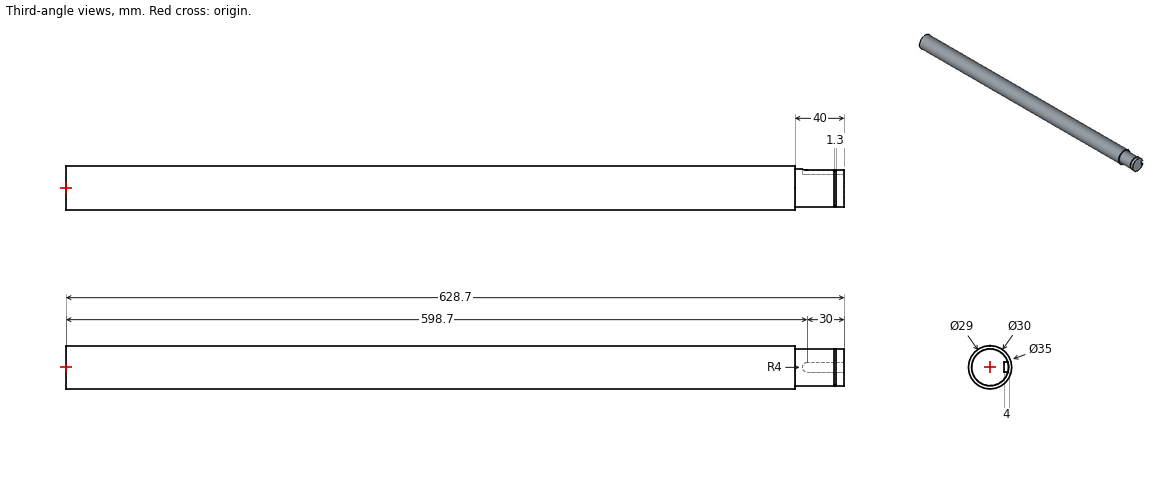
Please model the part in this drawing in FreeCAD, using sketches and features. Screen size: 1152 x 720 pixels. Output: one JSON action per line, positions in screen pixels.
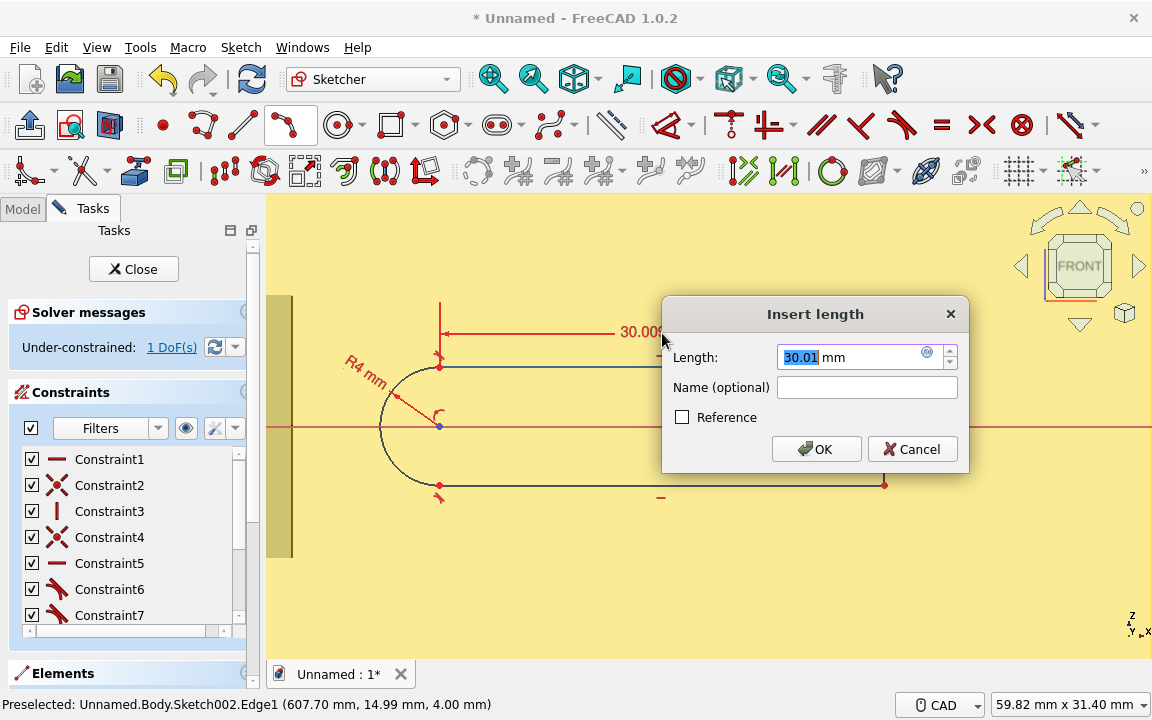
{"action": "type", "text": "30"}
{"action": "key", "text": "Return"}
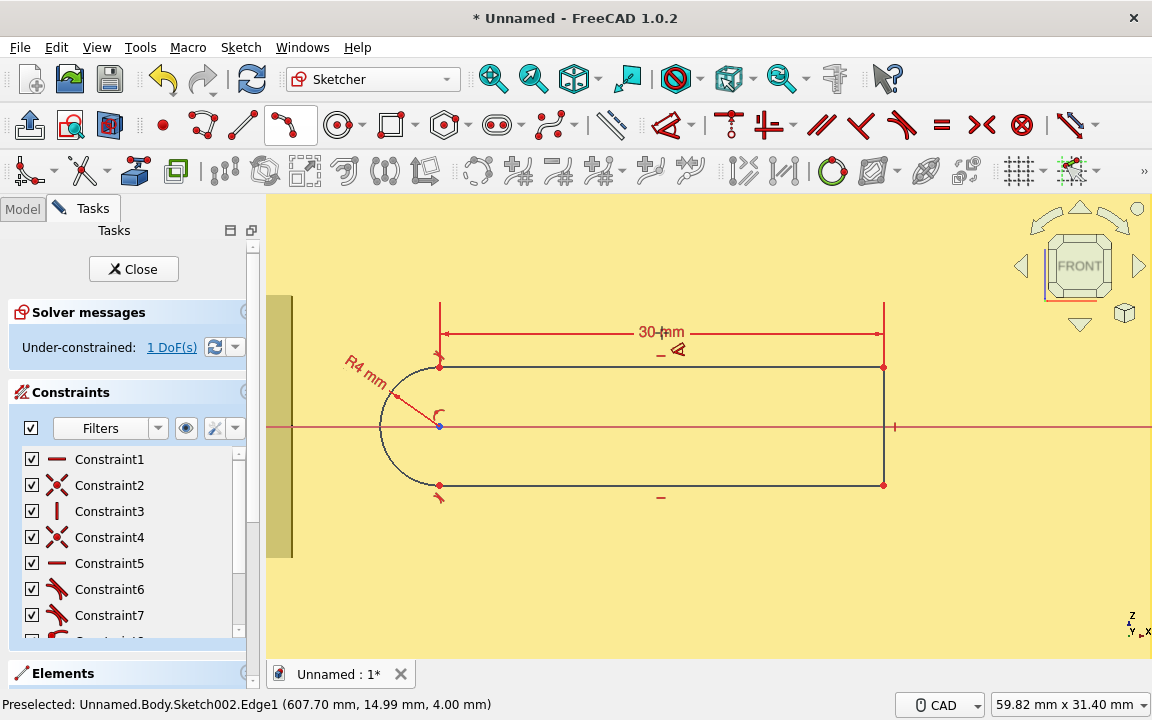
{"action": "left_click", "coordinate": [440, 367]}
{"action": "left_click", "coordinate": [367, 333]}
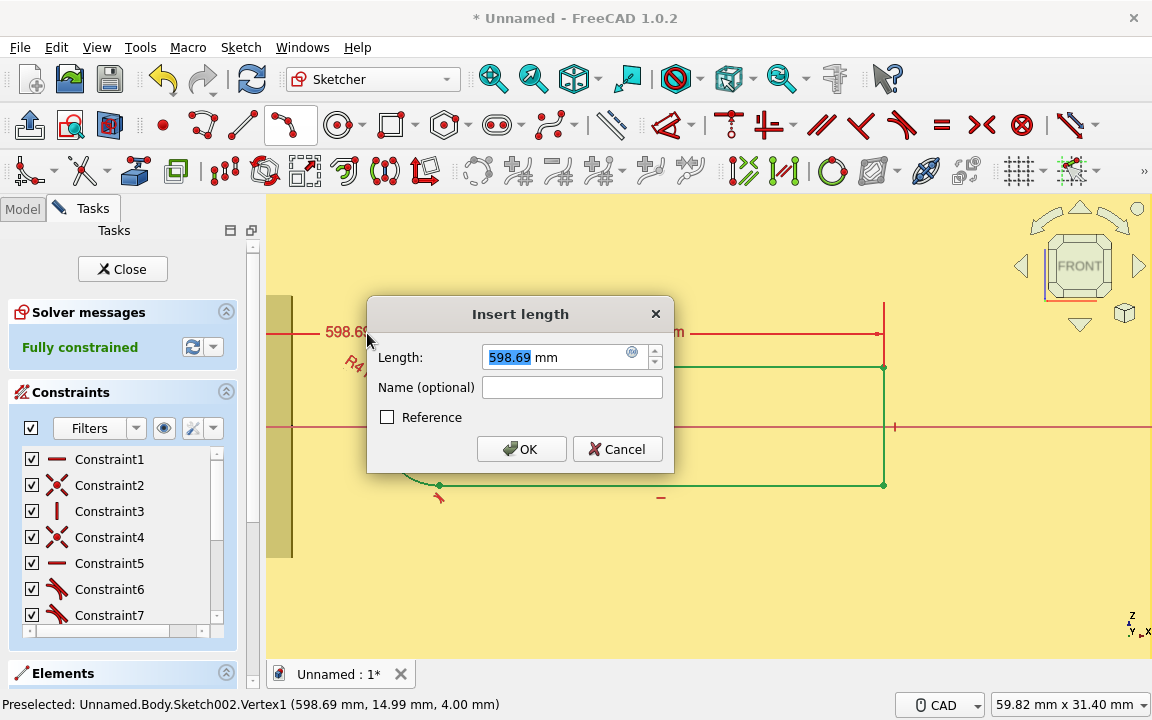
{"action": "type", "text": "598.7"}
{"action": "key", "text": "Return"}
{"action": "key", "text": "Escape"}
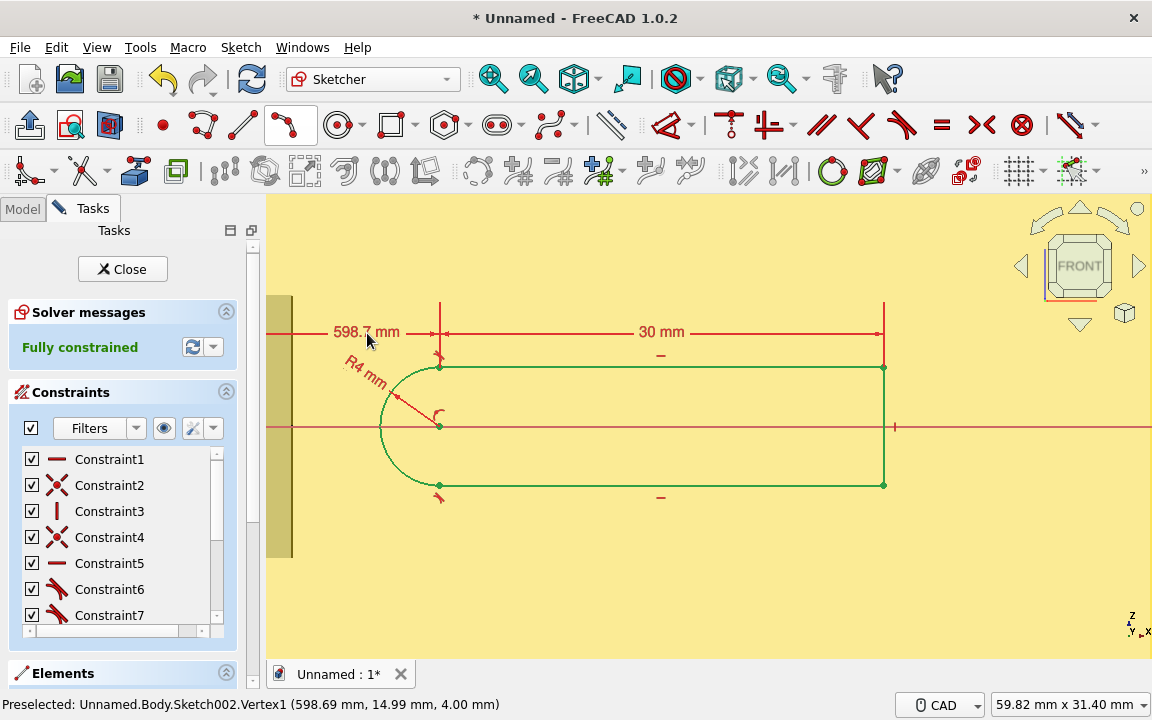
{"action": "left_click", "coordinate": [123, 269]}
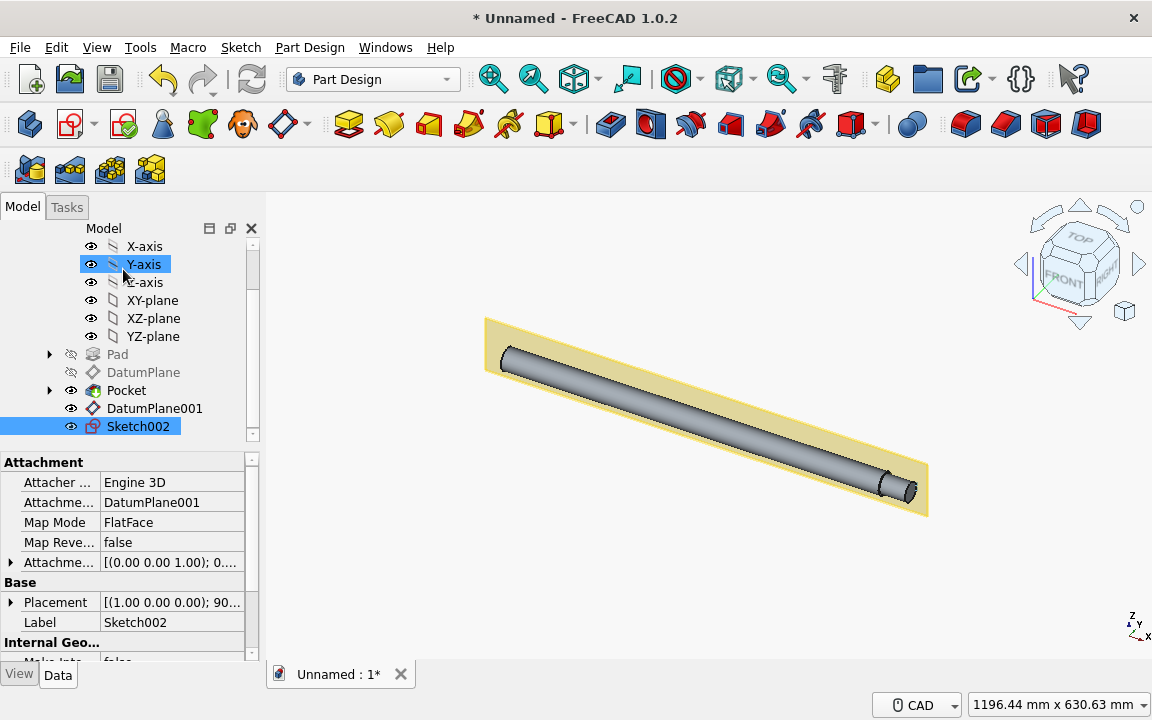
{"action": "left_click", "coordinate": [612, 124]}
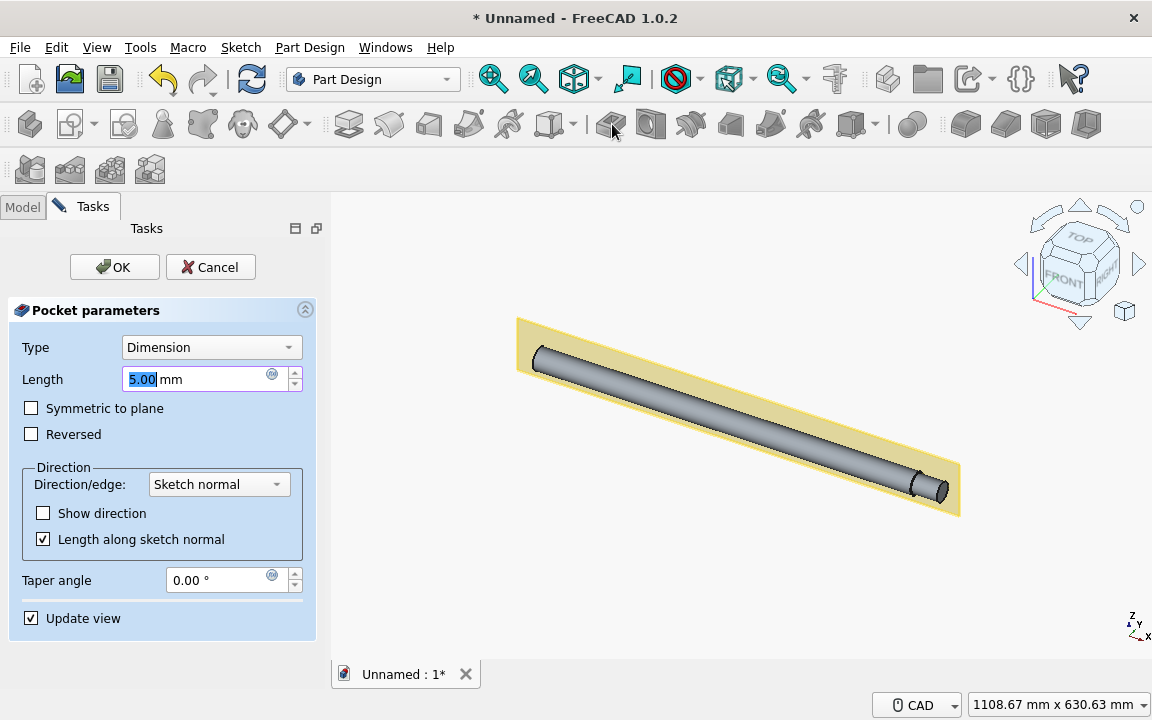
{"action": "type", "text": "4"}
{"action": "key", "text": "Tab"}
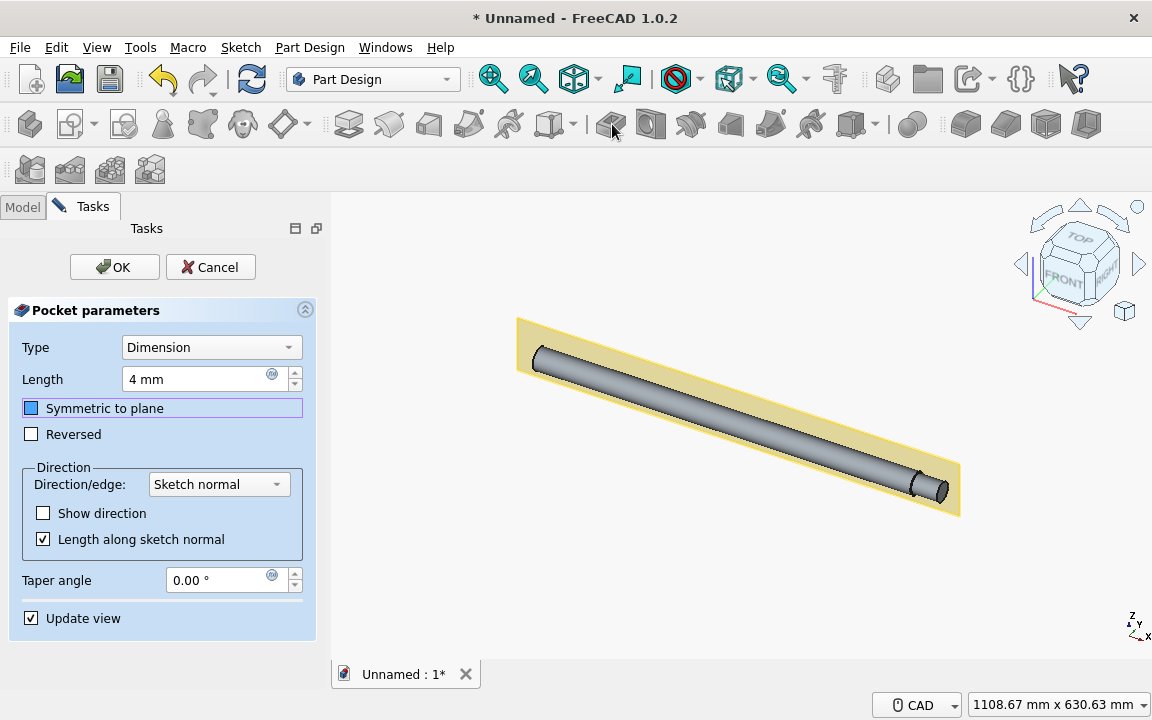
{"action": "left_click", "coordinate": [30, 434]}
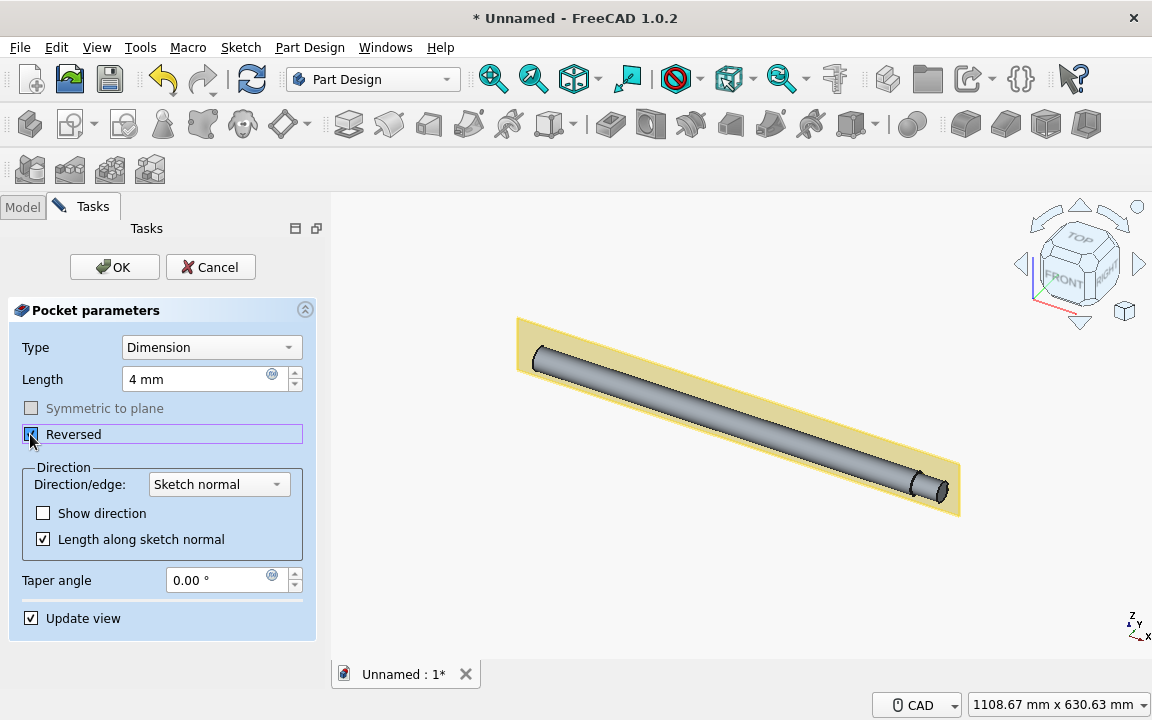
{"action": "left_click", "coordinate": [115, 267]}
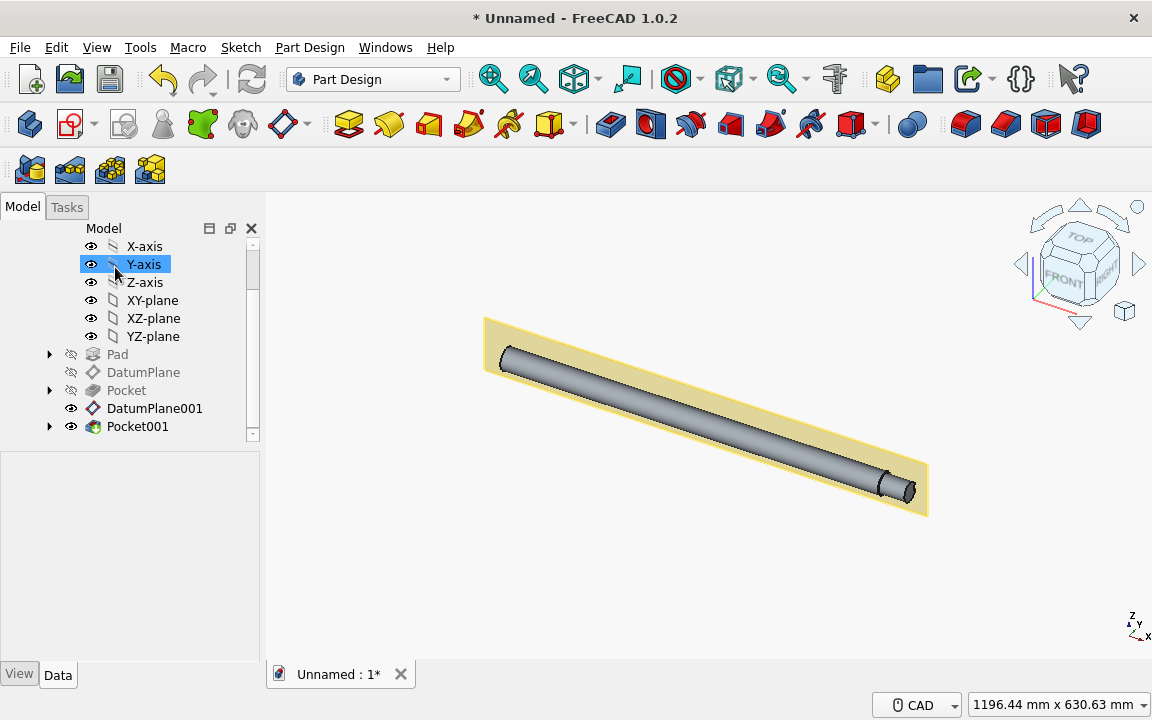
{"action": "left_click", "coordinate": [116, 408]}
{"action": "key", "text": "space"}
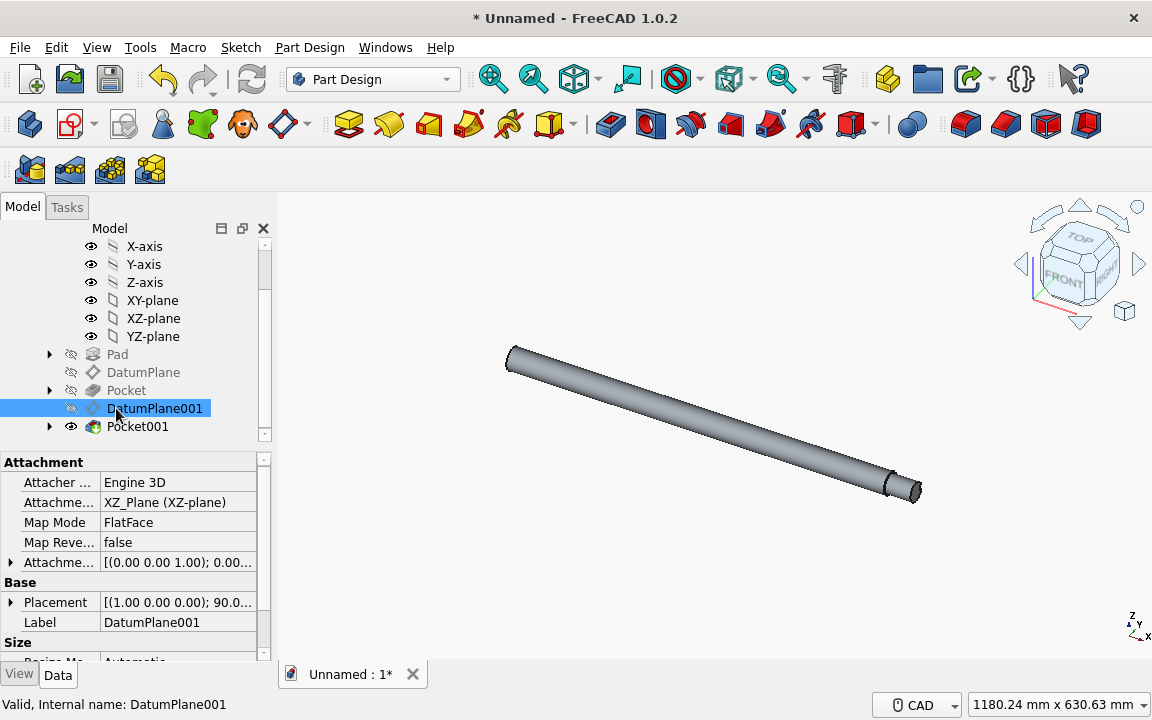
{"action": "scroll", "coordinate": [160, 332], "scroll_direction": "down", "scroll_amount": 3}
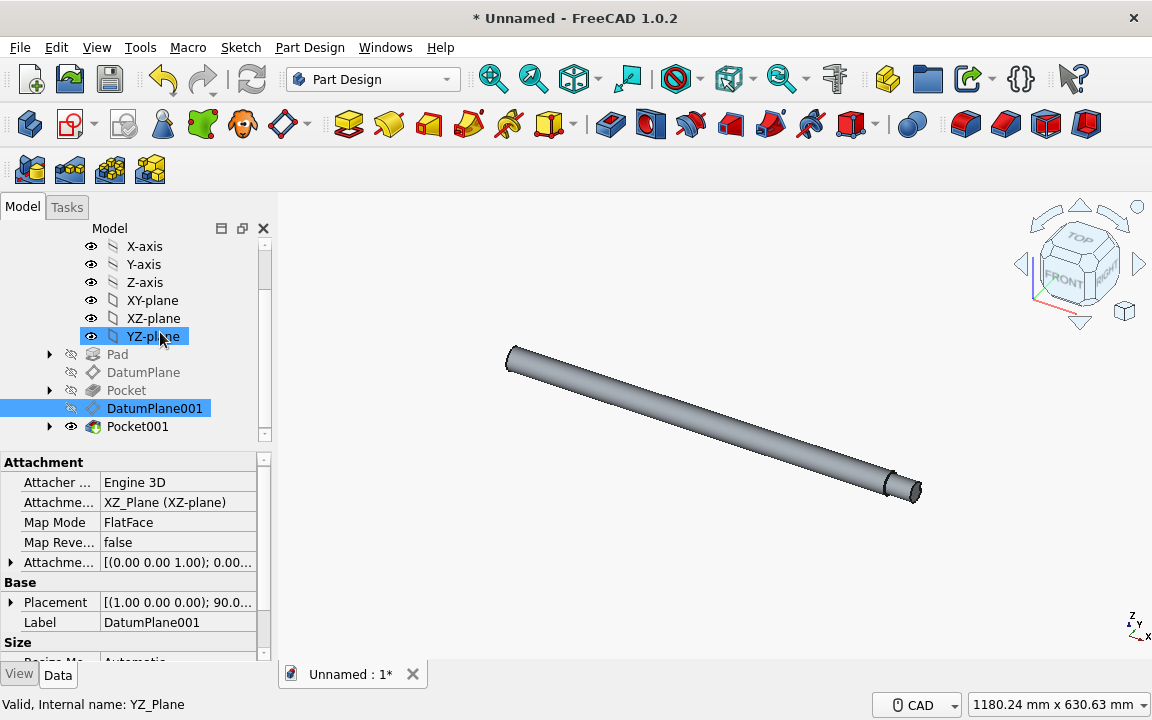
{"action": "scroll", "coordinate": [160, 332], "scroll_direction": "up", "scroll_amount": 15}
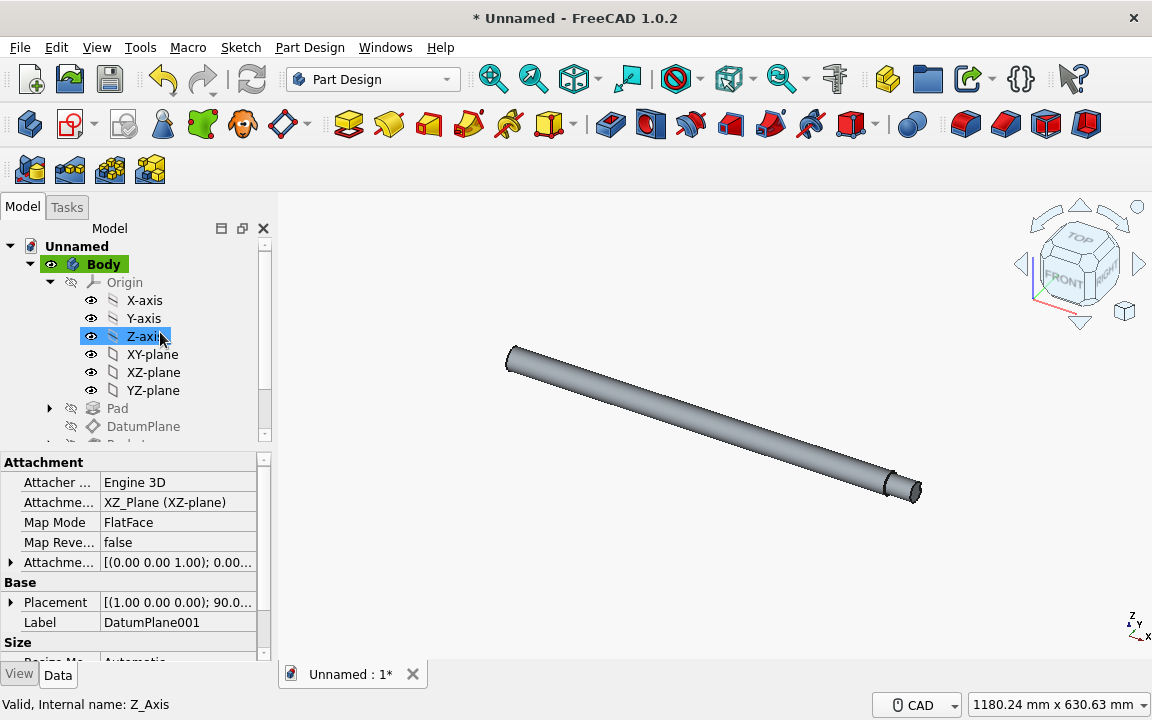
{"action": "left_click", "coordinate": [136, 390]}